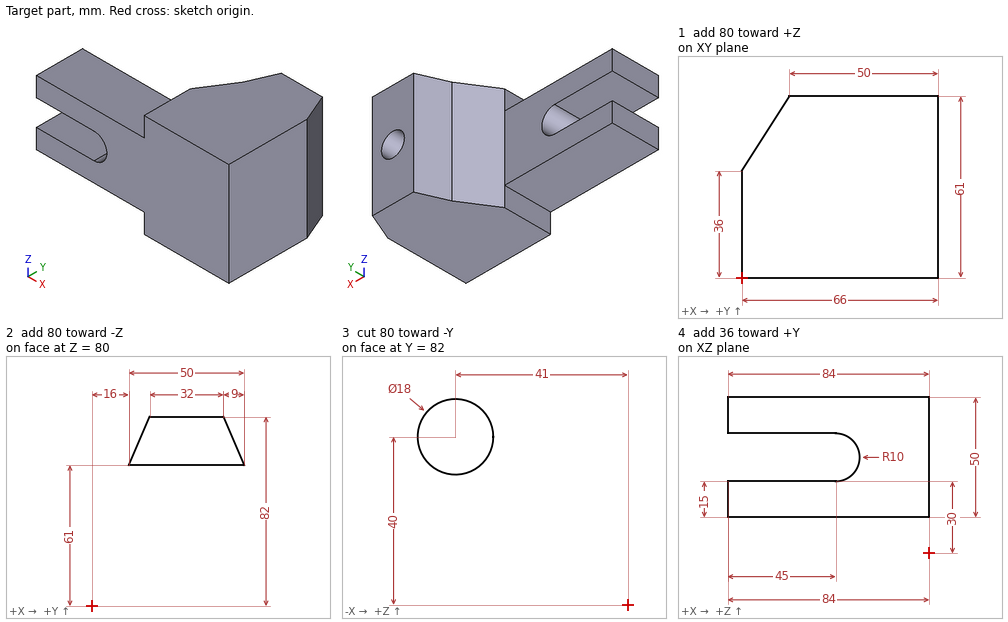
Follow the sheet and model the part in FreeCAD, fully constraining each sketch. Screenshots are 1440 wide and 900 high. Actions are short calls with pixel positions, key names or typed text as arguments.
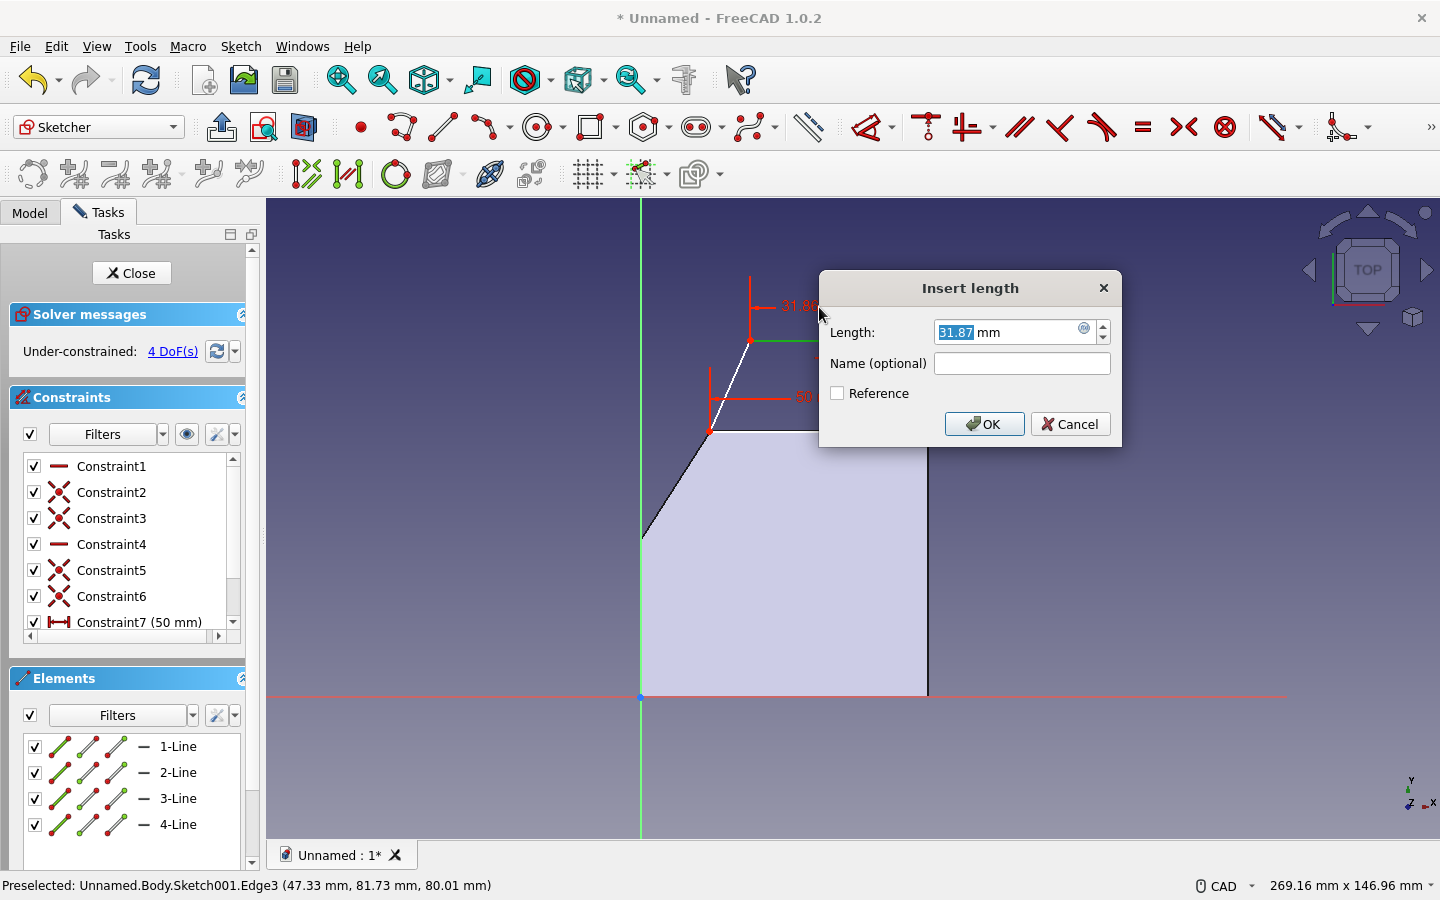
text(32)
key(Return)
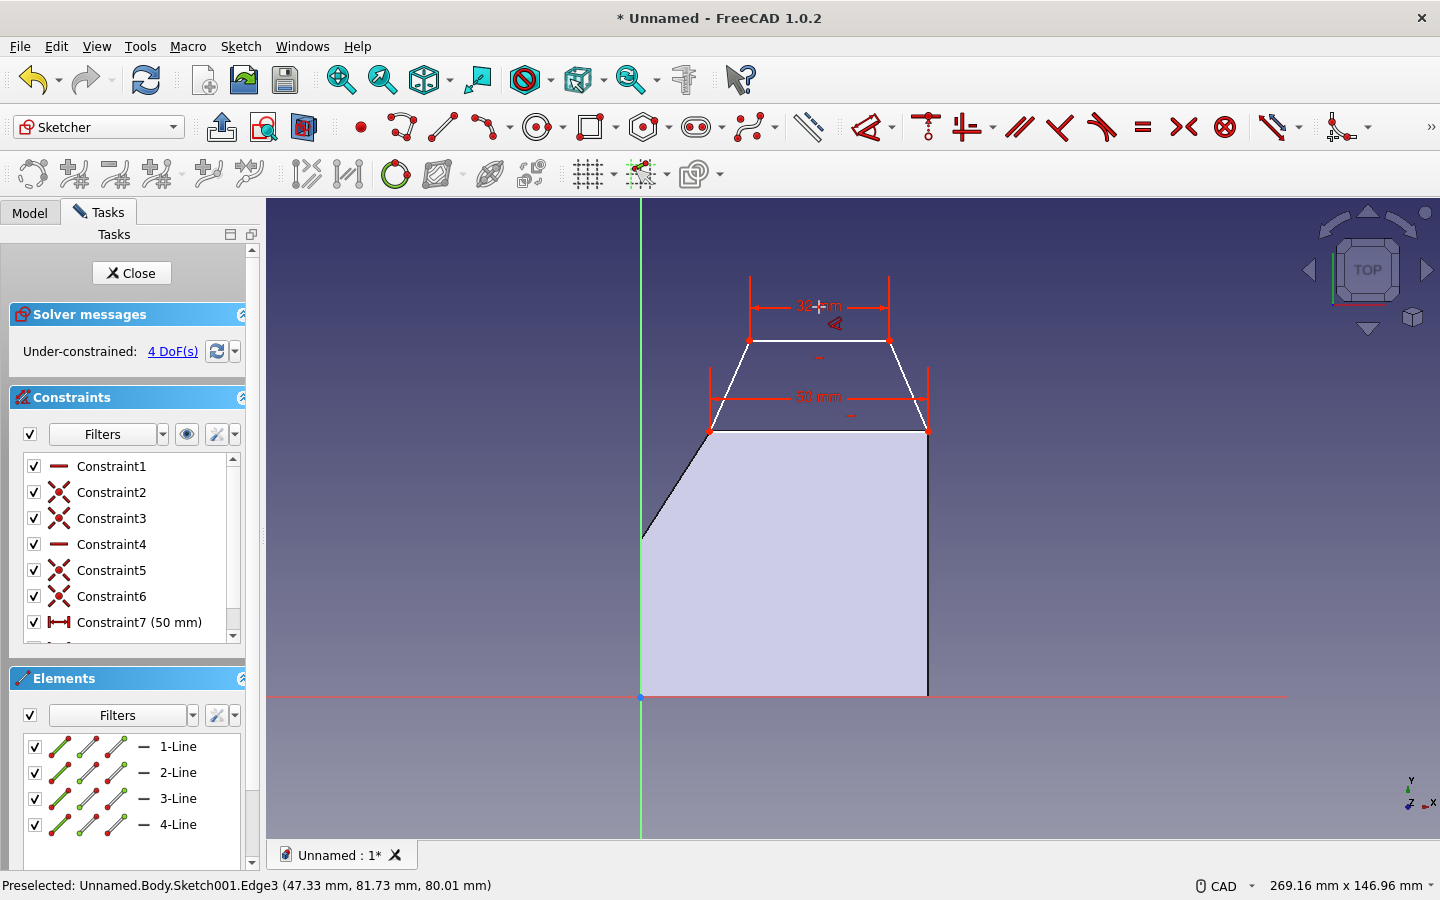
click(916, 405)
click(909, 307)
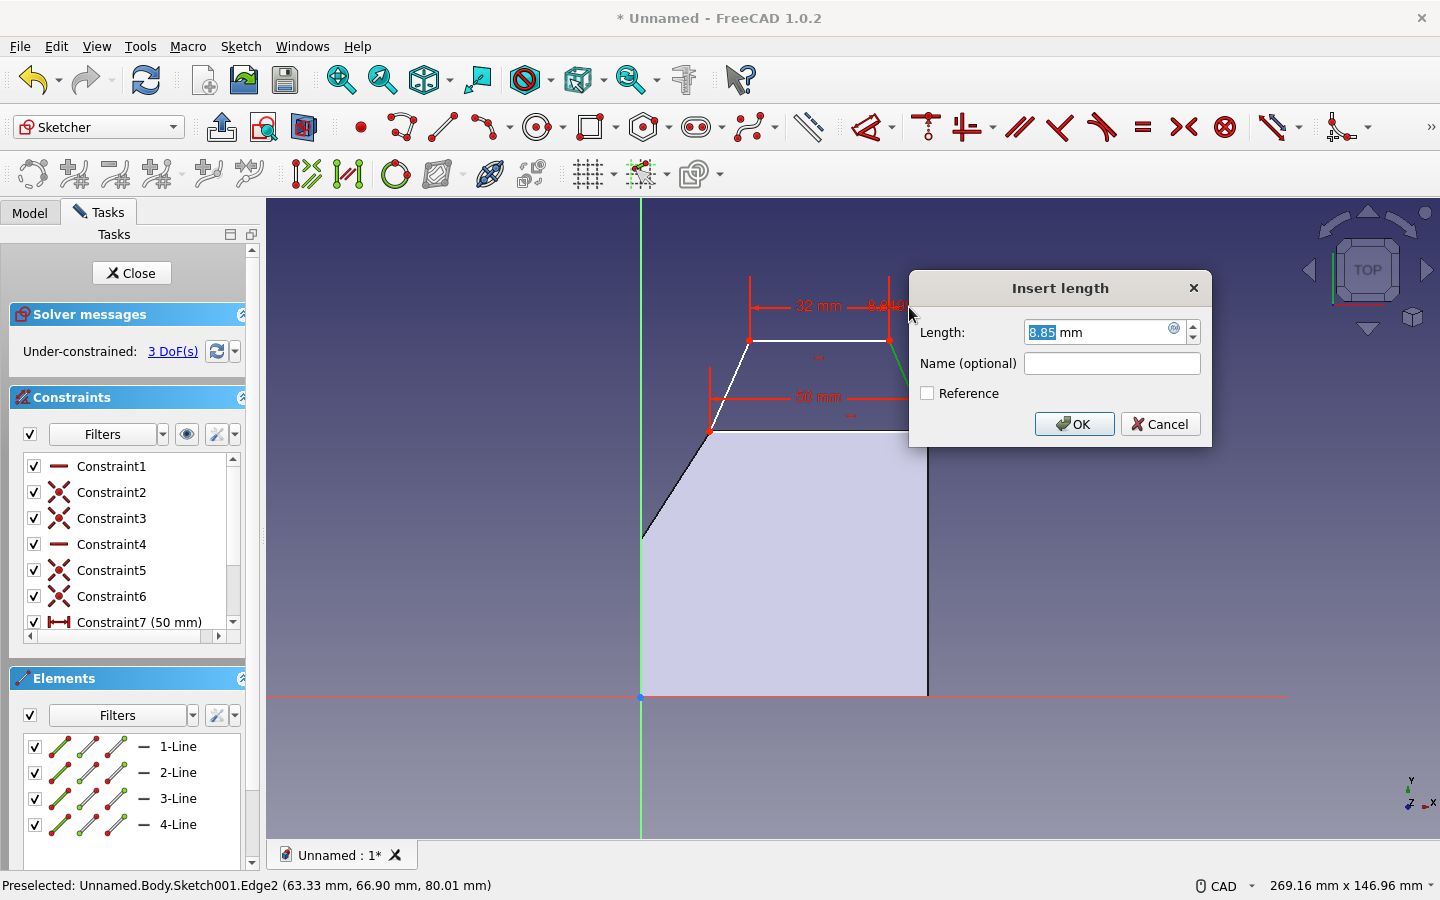
text(9)
key(Return)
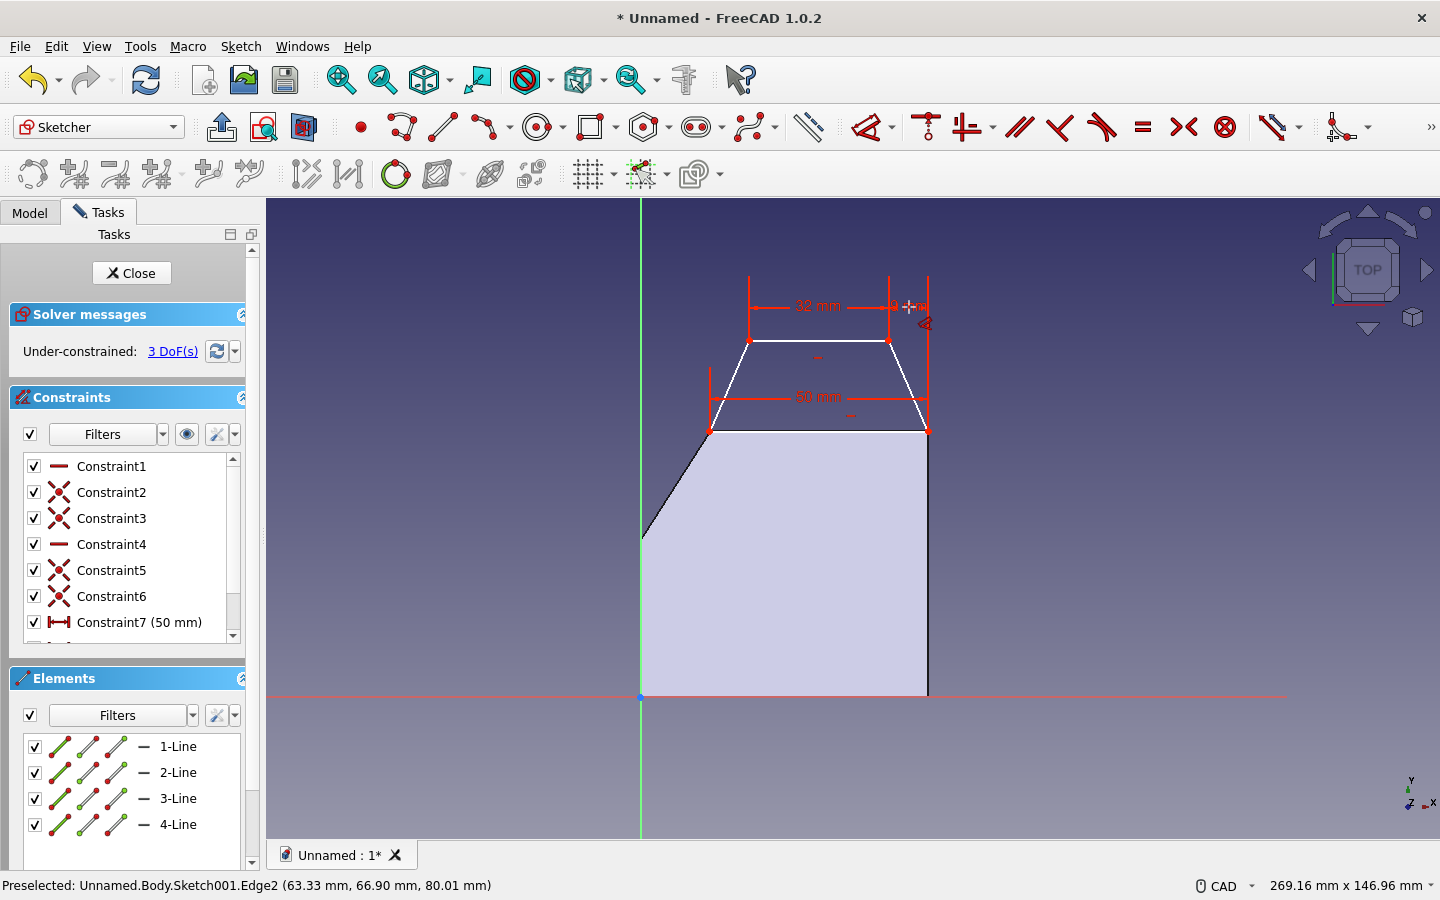
click(710, 432)
click(675, 731)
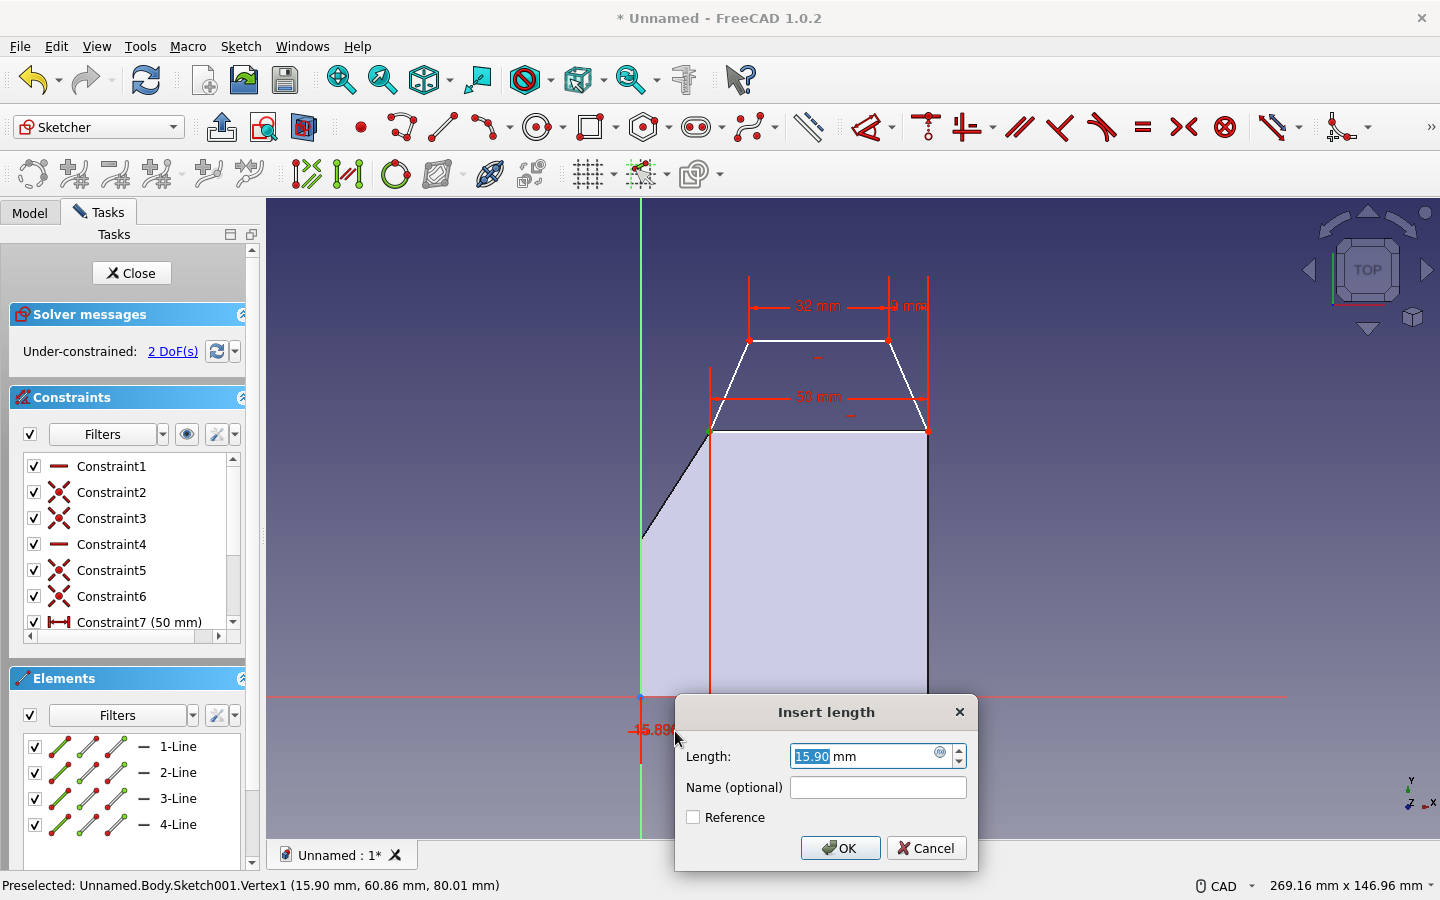
text(16)
key(Return)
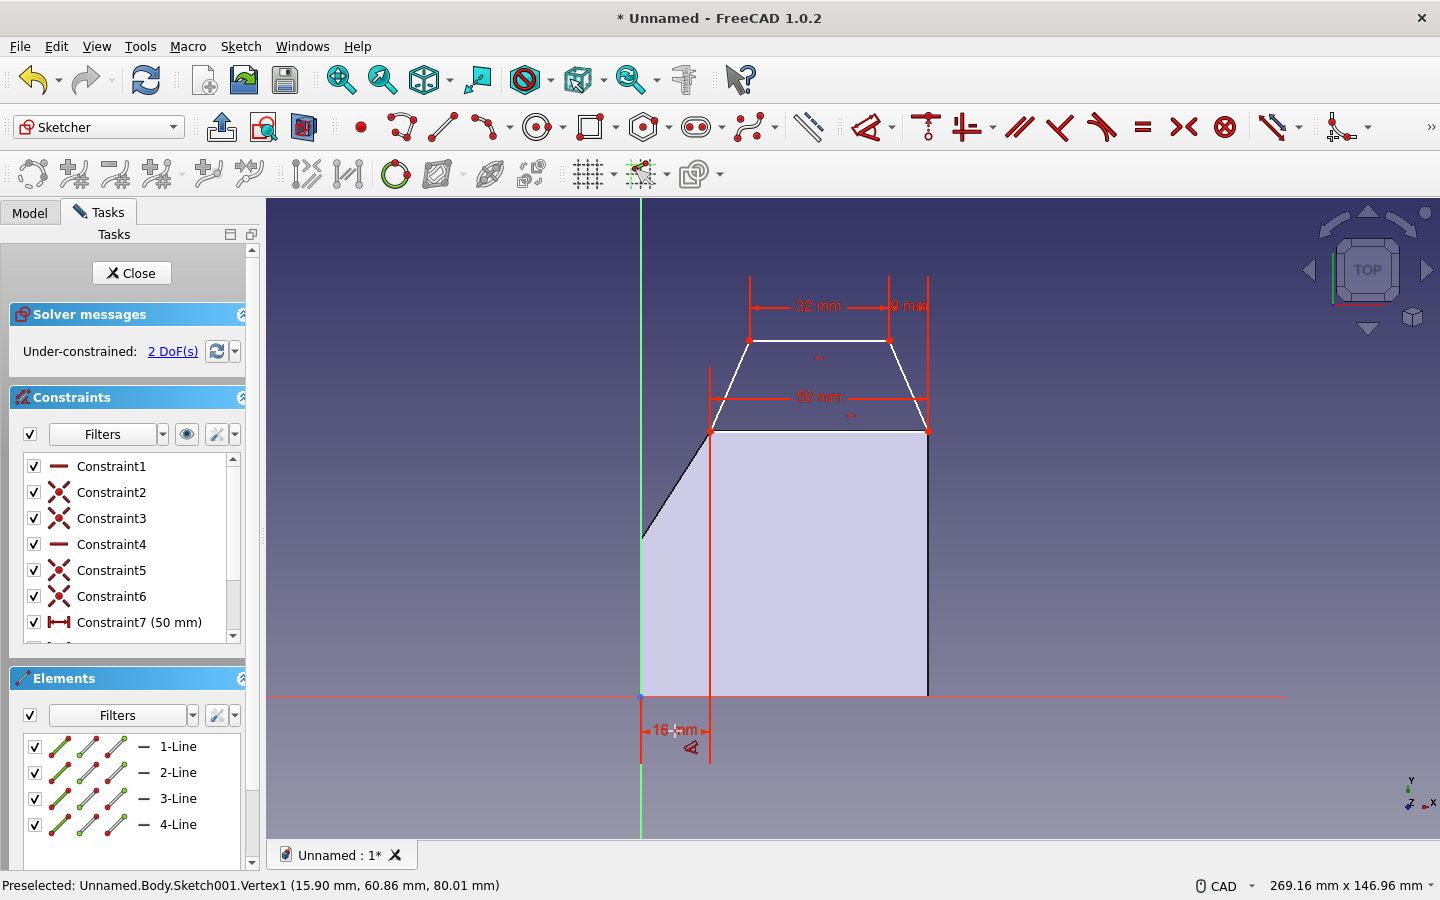
click(710, 432)
click(607, 565)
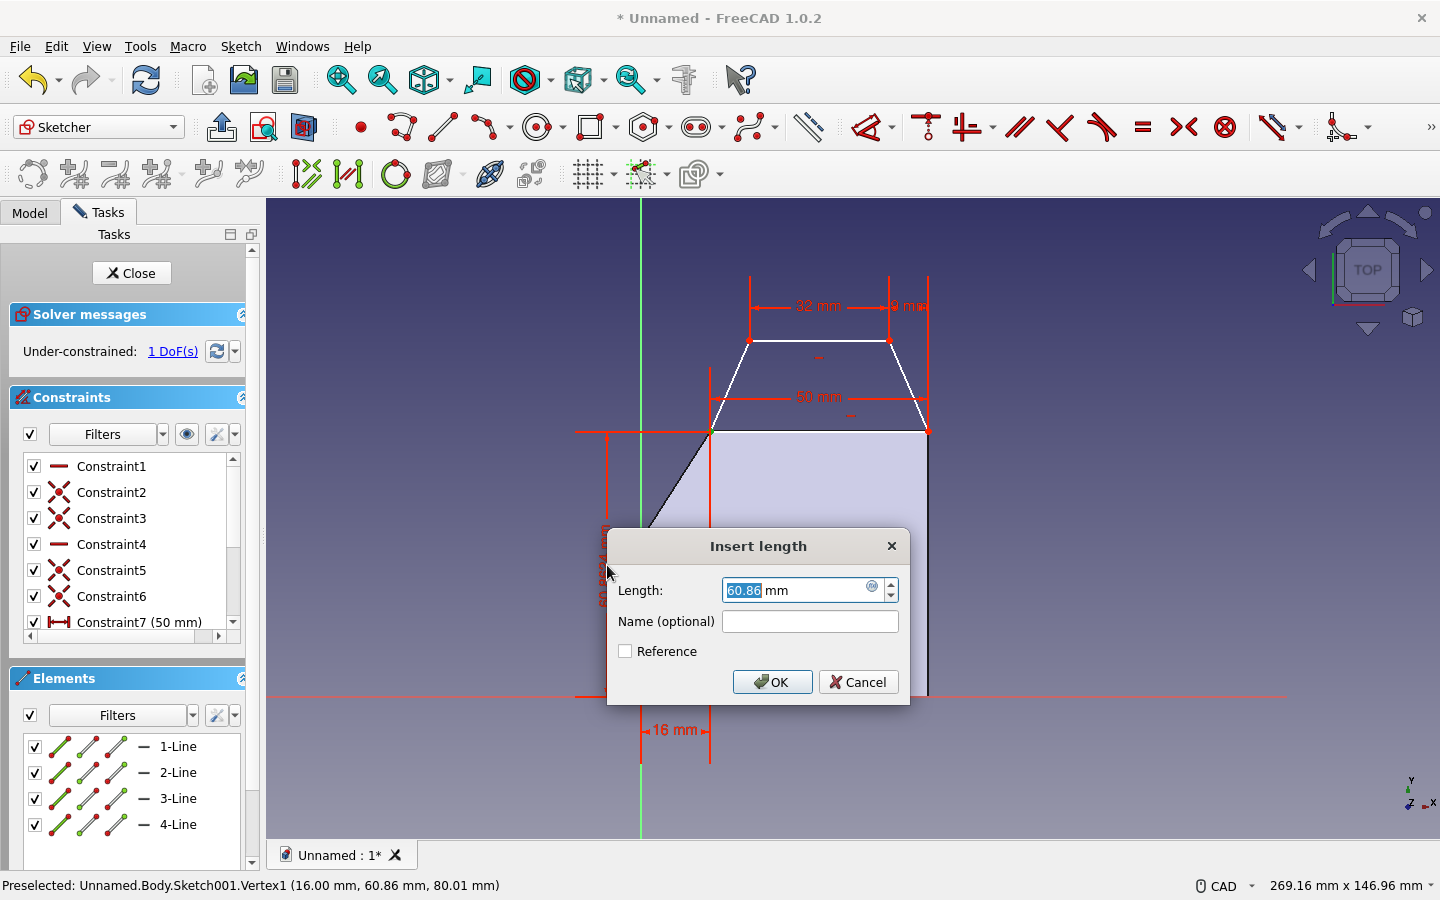
text(61)
key(Return)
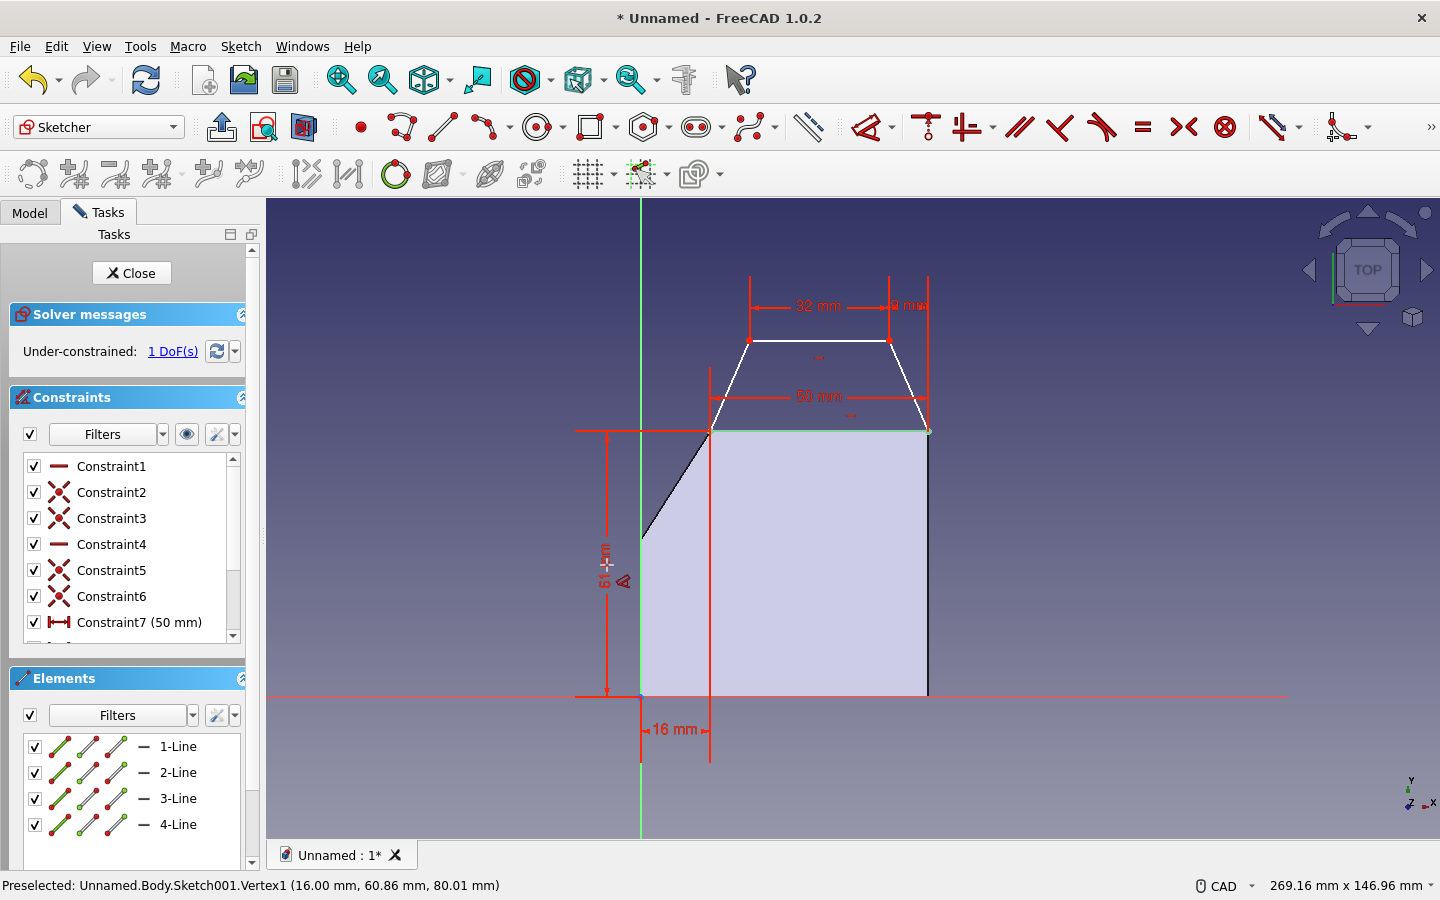
click(889, 341)
click(607, 519)